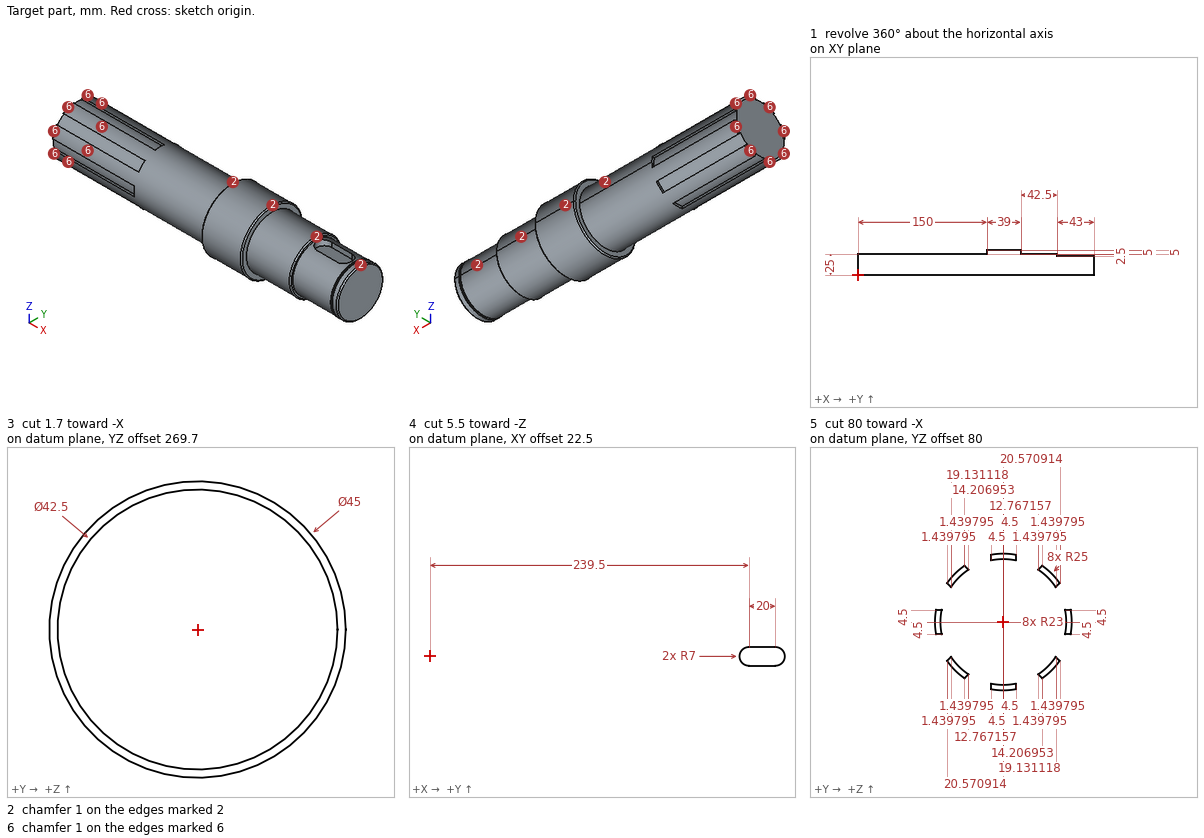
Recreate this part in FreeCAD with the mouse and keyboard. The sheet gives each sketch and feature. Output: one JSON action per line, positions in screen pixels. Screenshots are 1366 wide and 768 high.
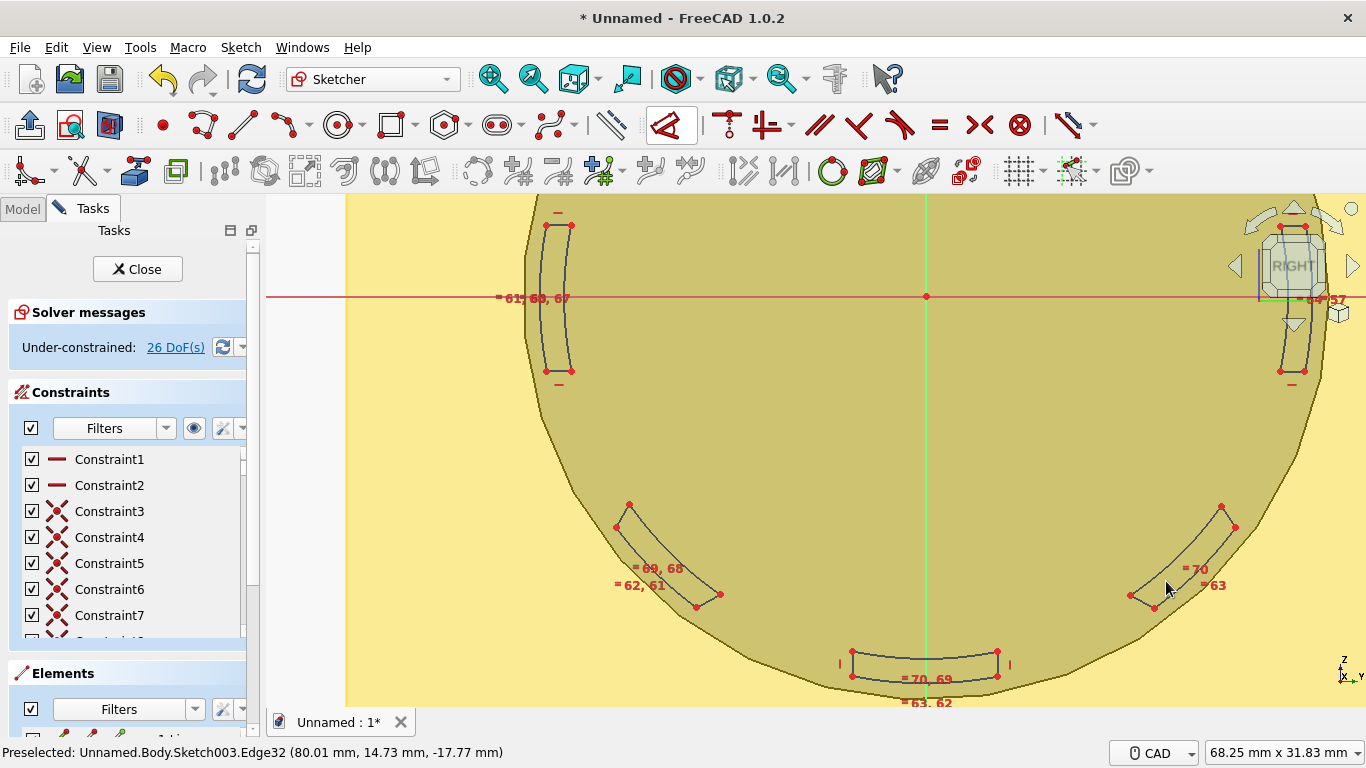
{"action": "scroll", "coordinate": [644, 540], "scroll_direction": "down", "scroll_amount": 5}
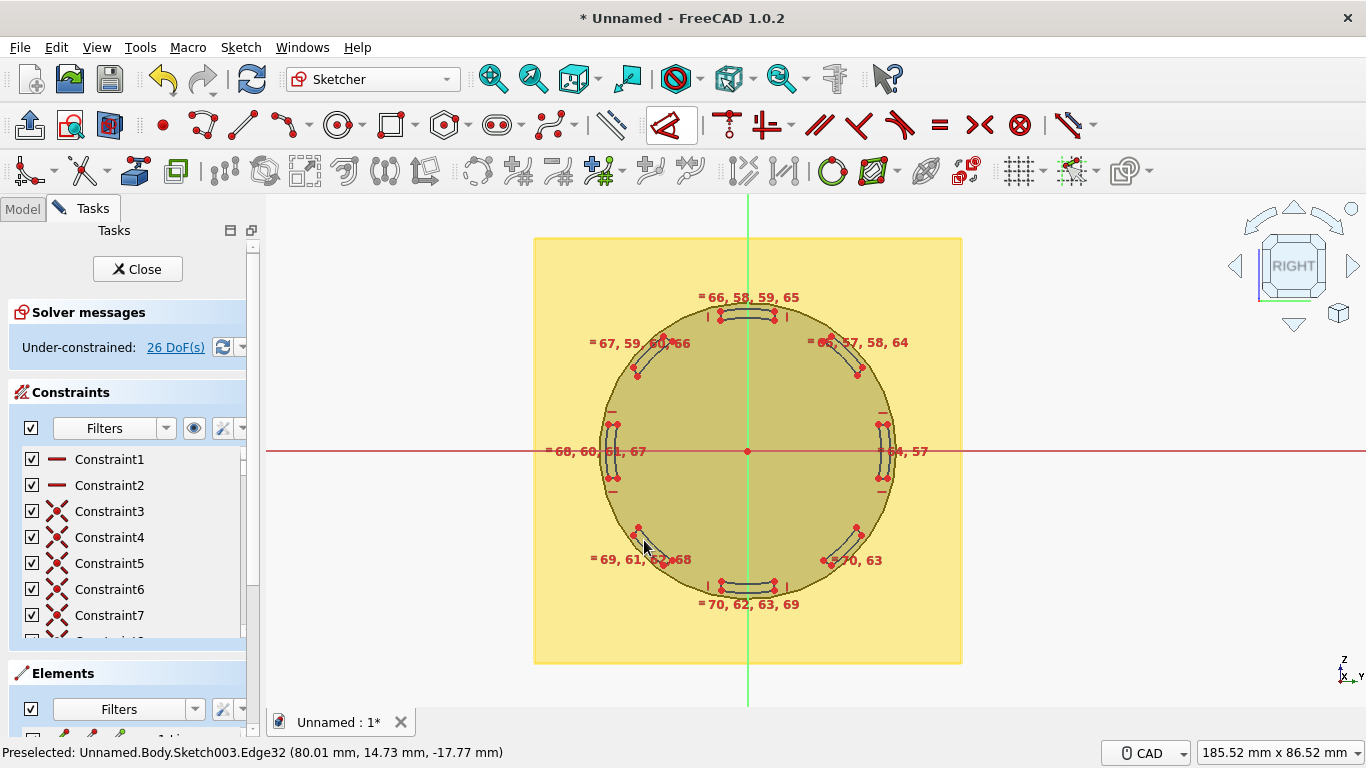
{"action": "scroll", "coordinate": [881, 463], "scroll_direction": "up", "scroll_amount": 3}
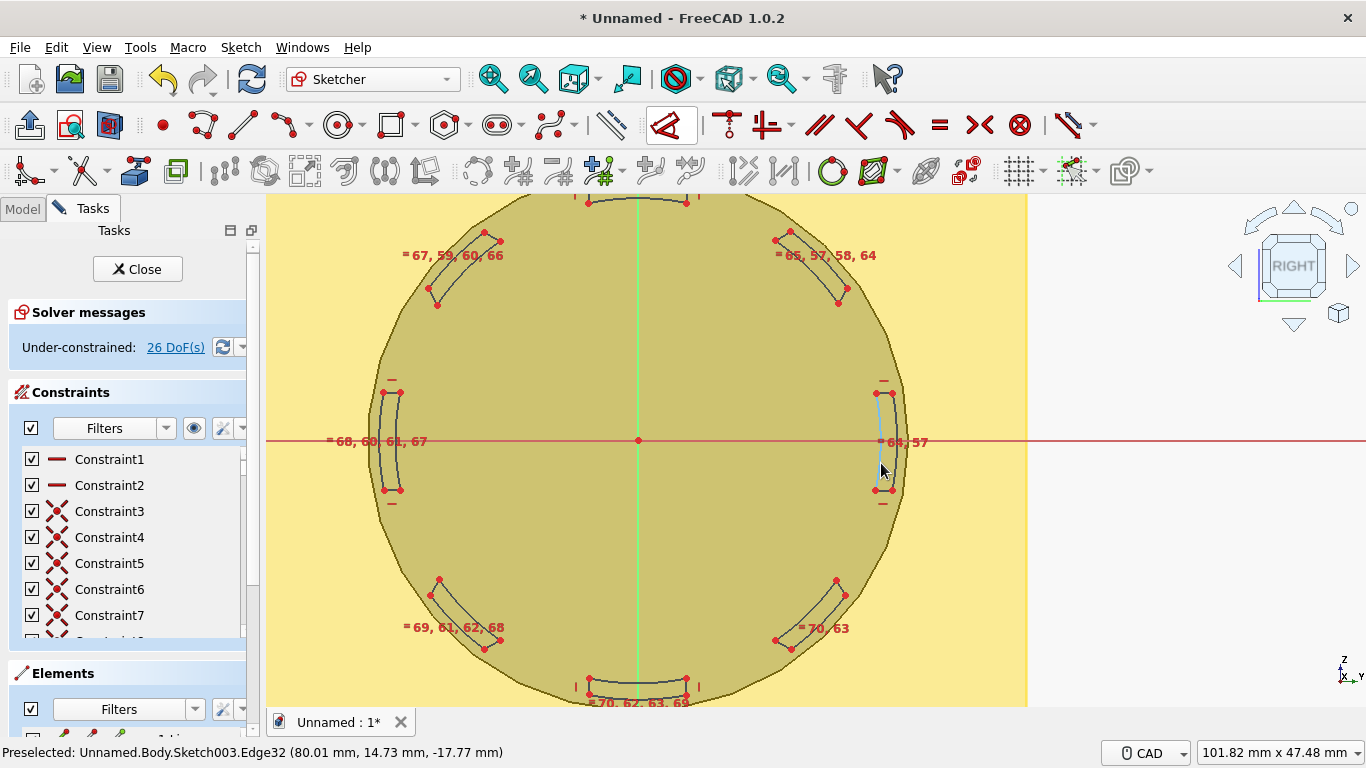
{"action": "left_click", "coordinate": [880, 462]}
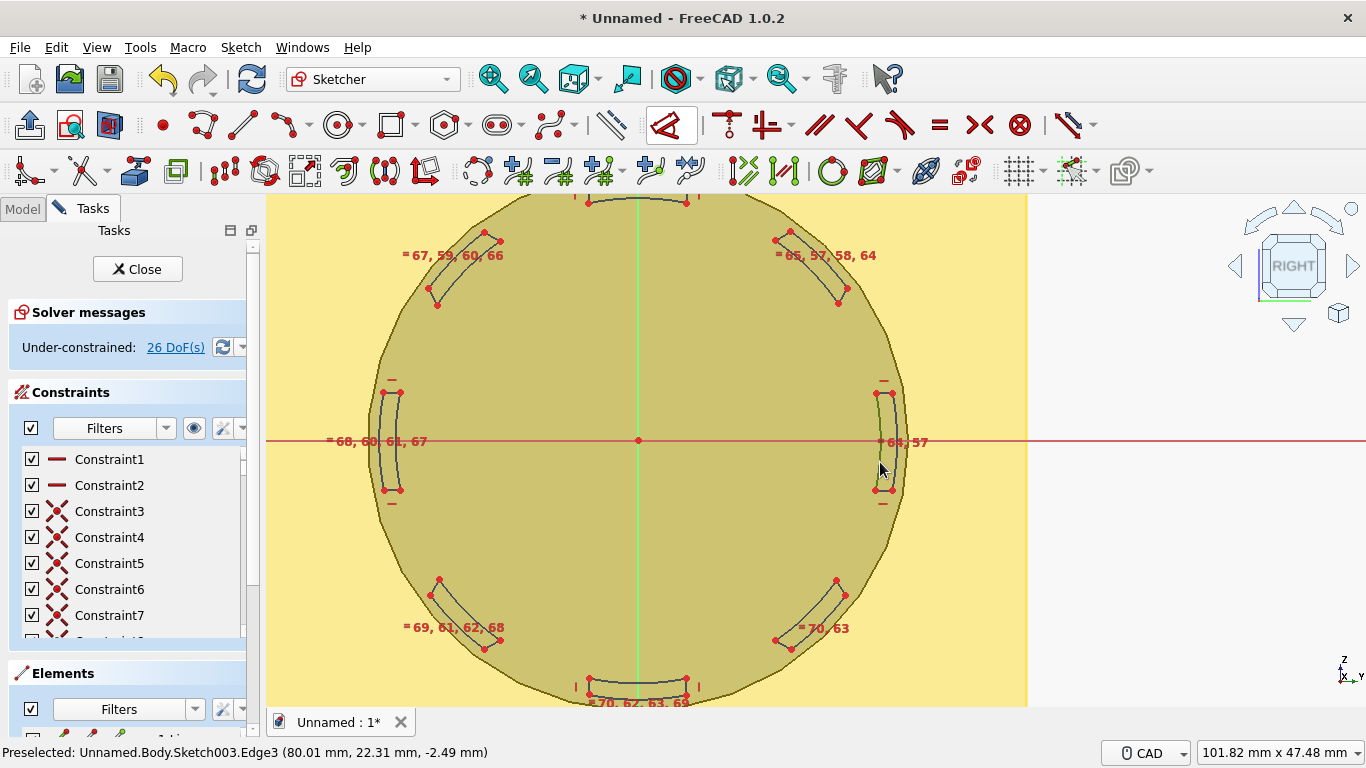
{"action": "left_click", "coordinate": [692, 126]}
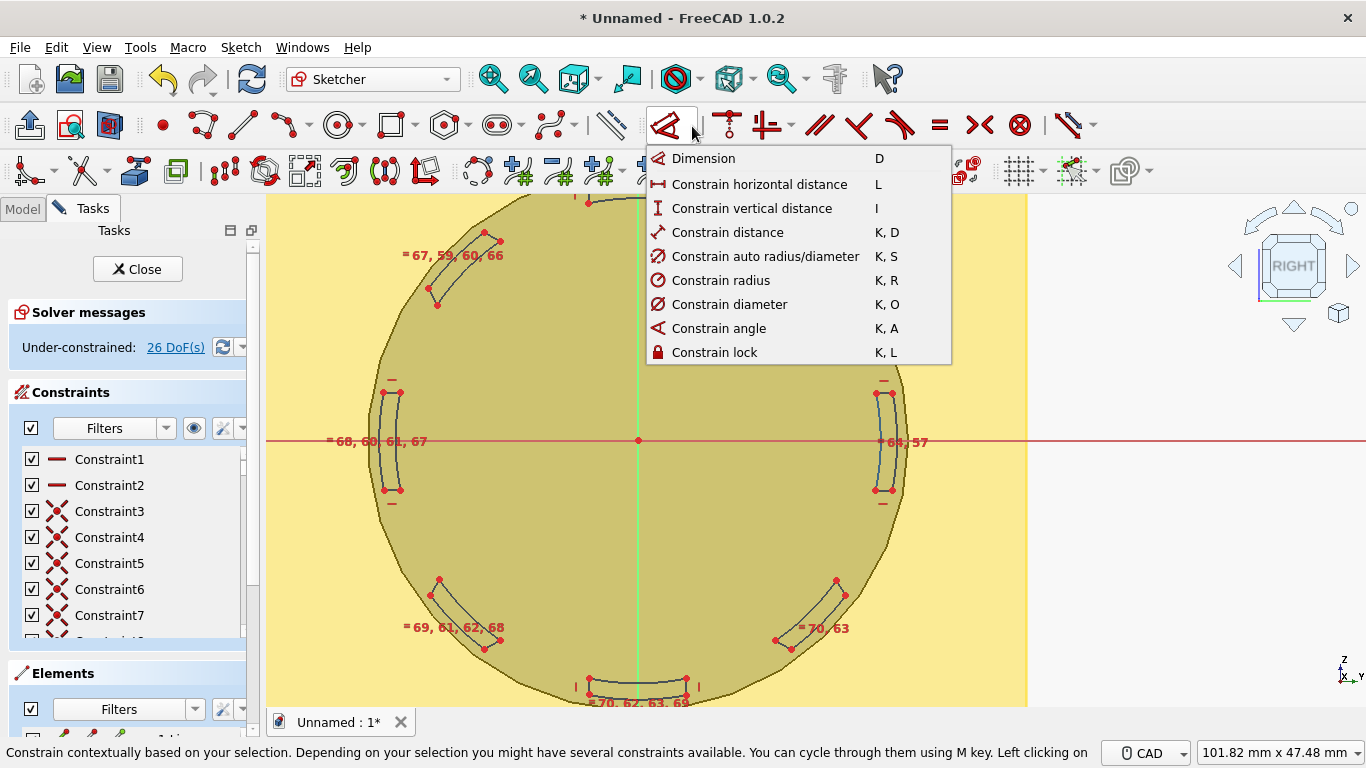
{"action": "left_click", "coordinate": [799, 280]}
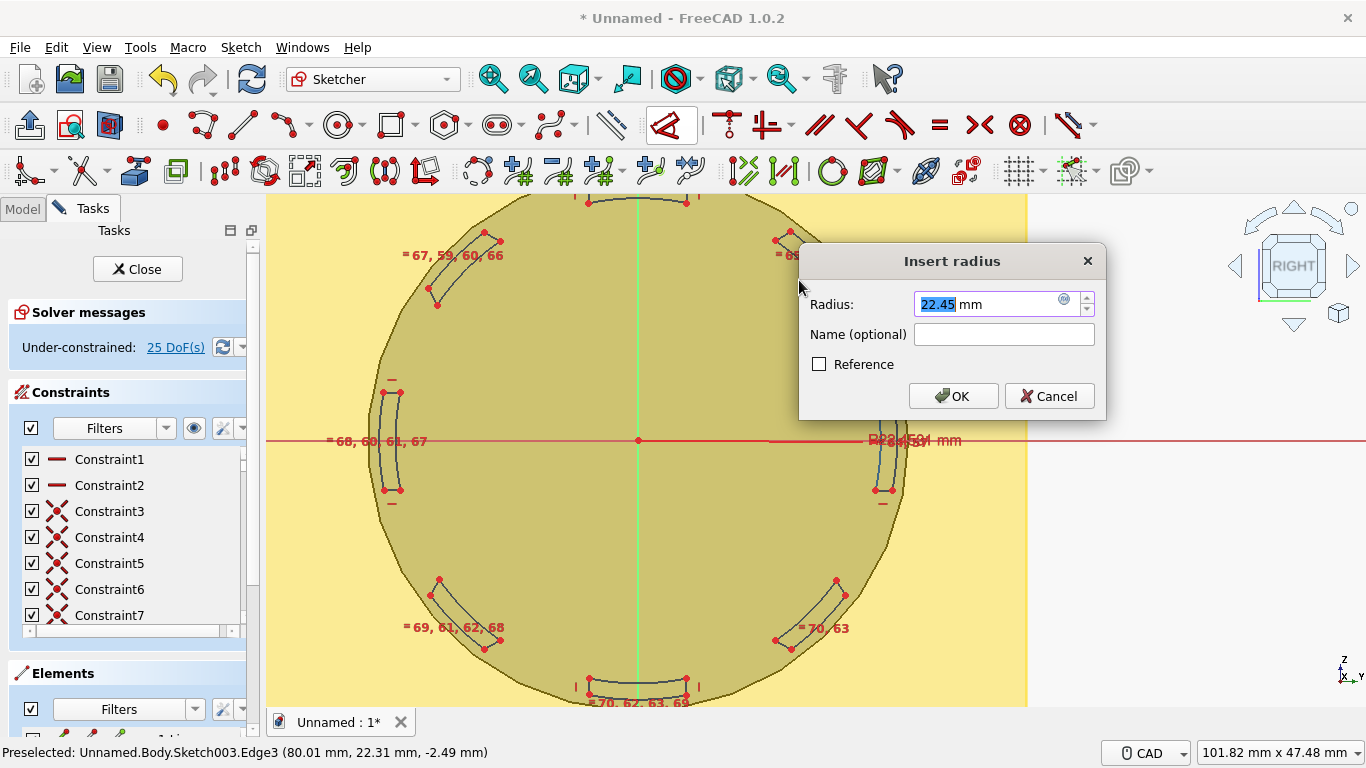
{"action": "type", "text": "23"}
{"action": "key", "text": "Return"}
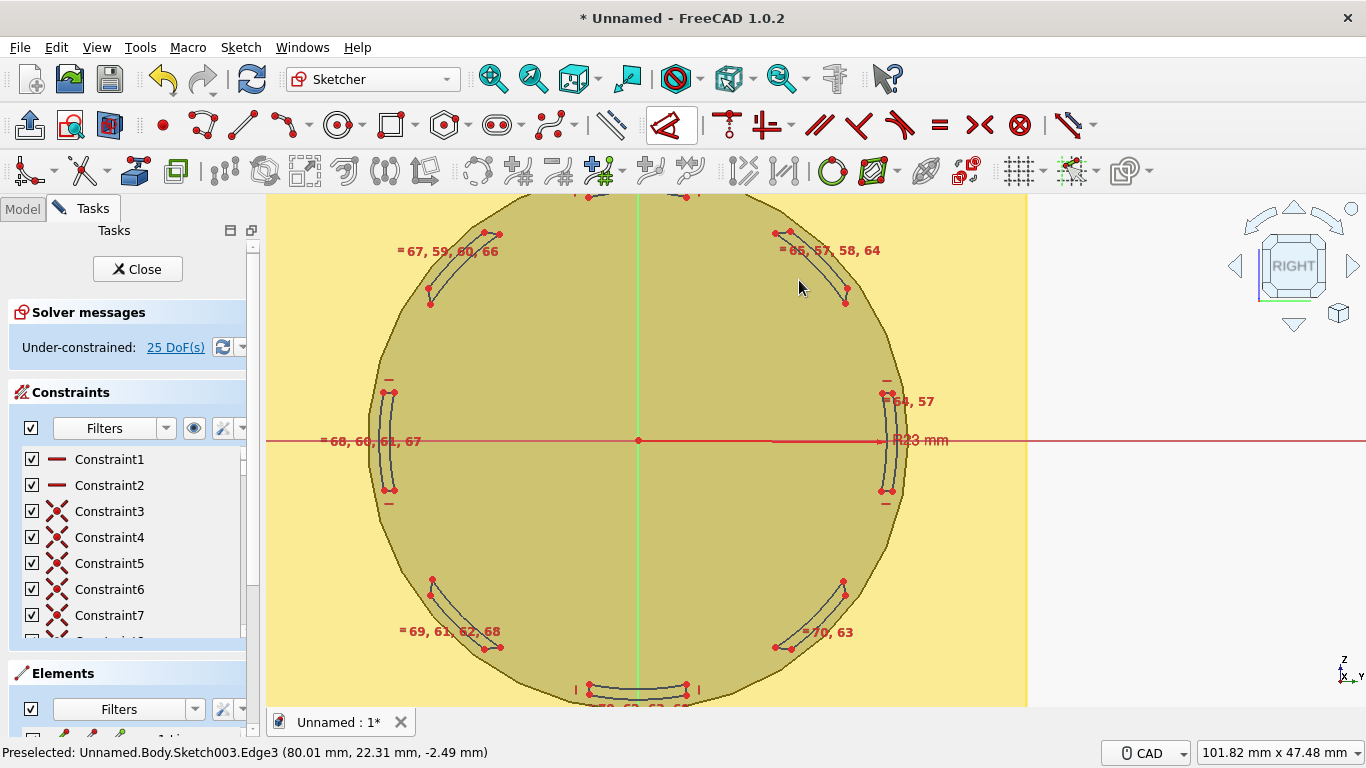
{"action": "scroll", "coordinate": [896, 462], "scroll_direction": "up", "scroll_amount": 2}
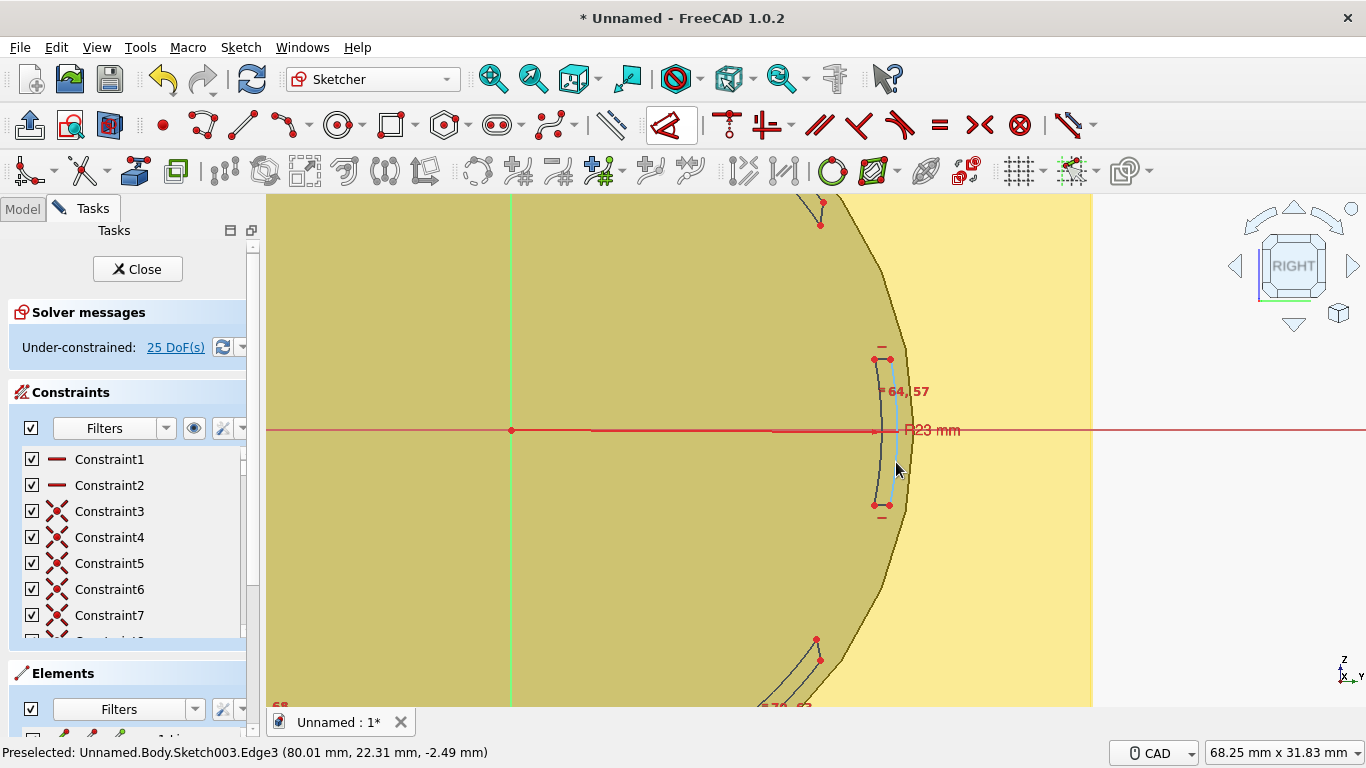
{"action": "left_click", "coordinate": [896, 461]}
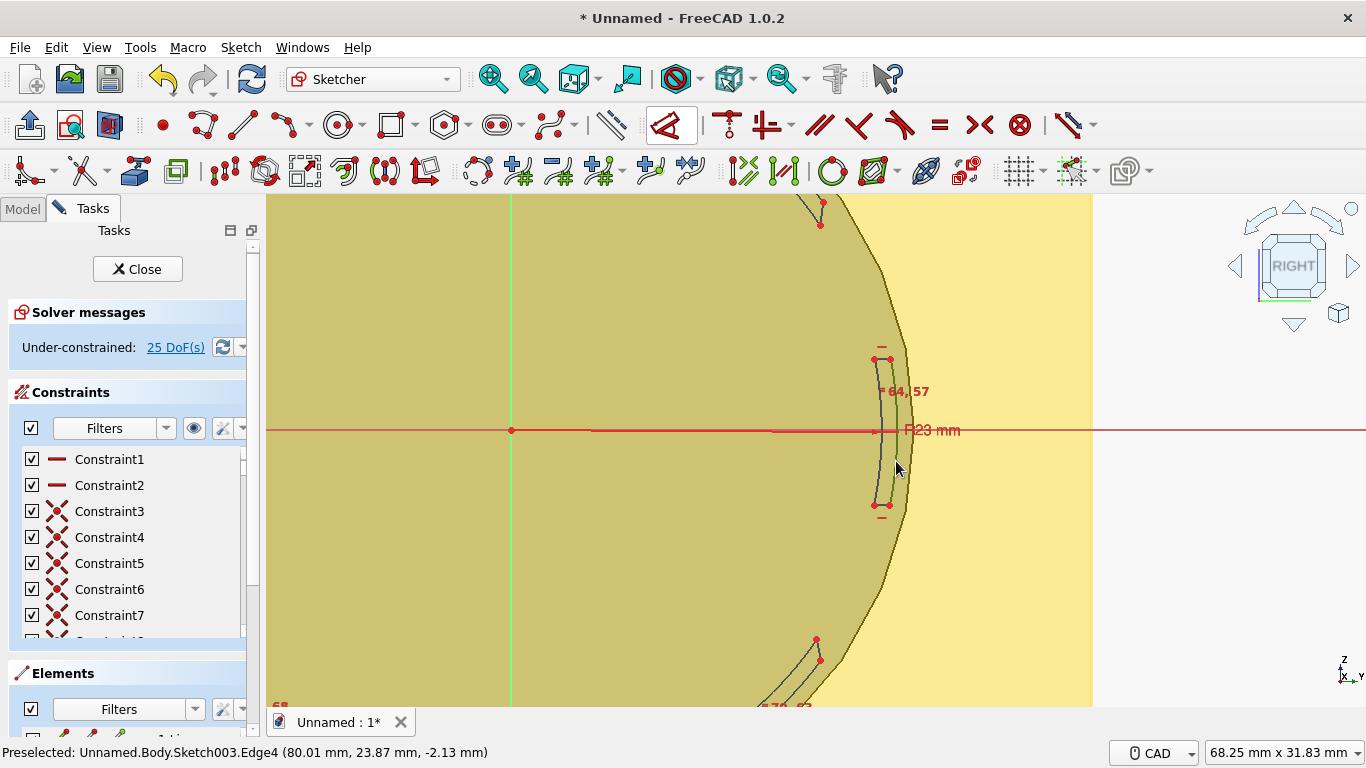
{"action": "key", "text": "k r"}